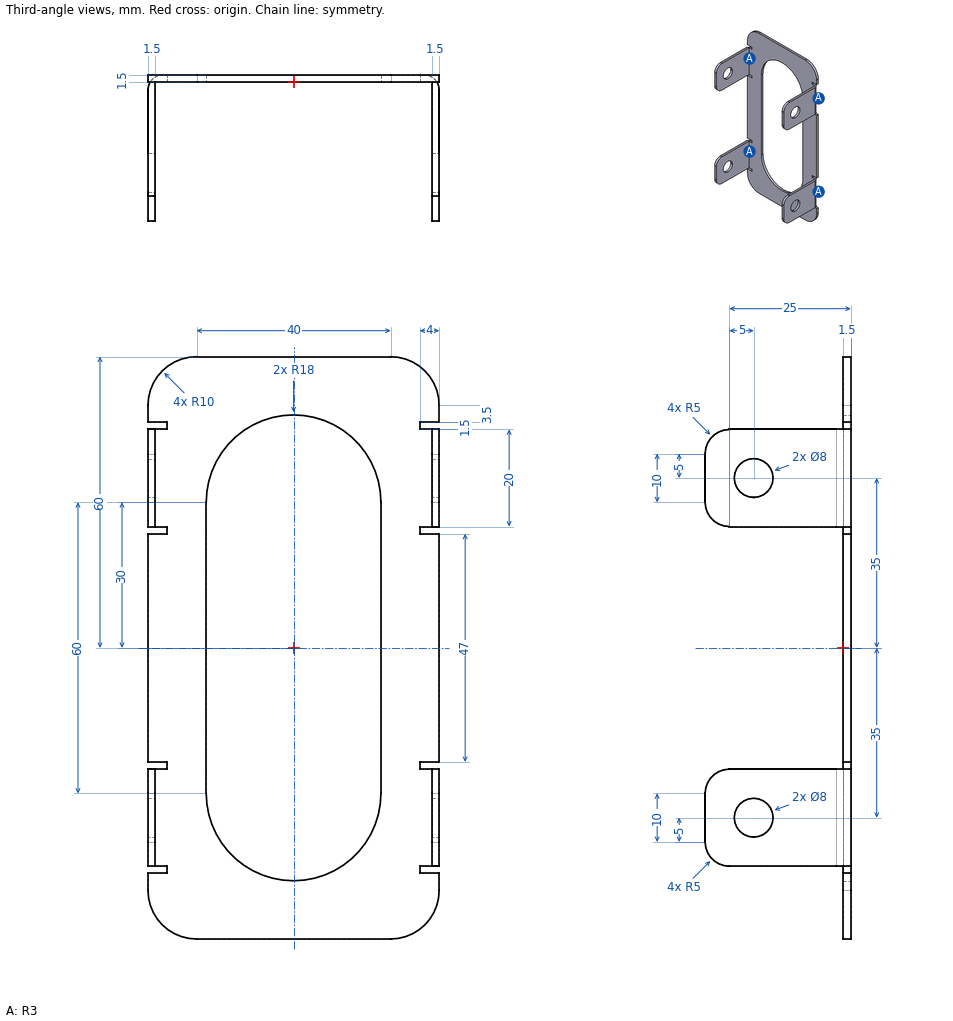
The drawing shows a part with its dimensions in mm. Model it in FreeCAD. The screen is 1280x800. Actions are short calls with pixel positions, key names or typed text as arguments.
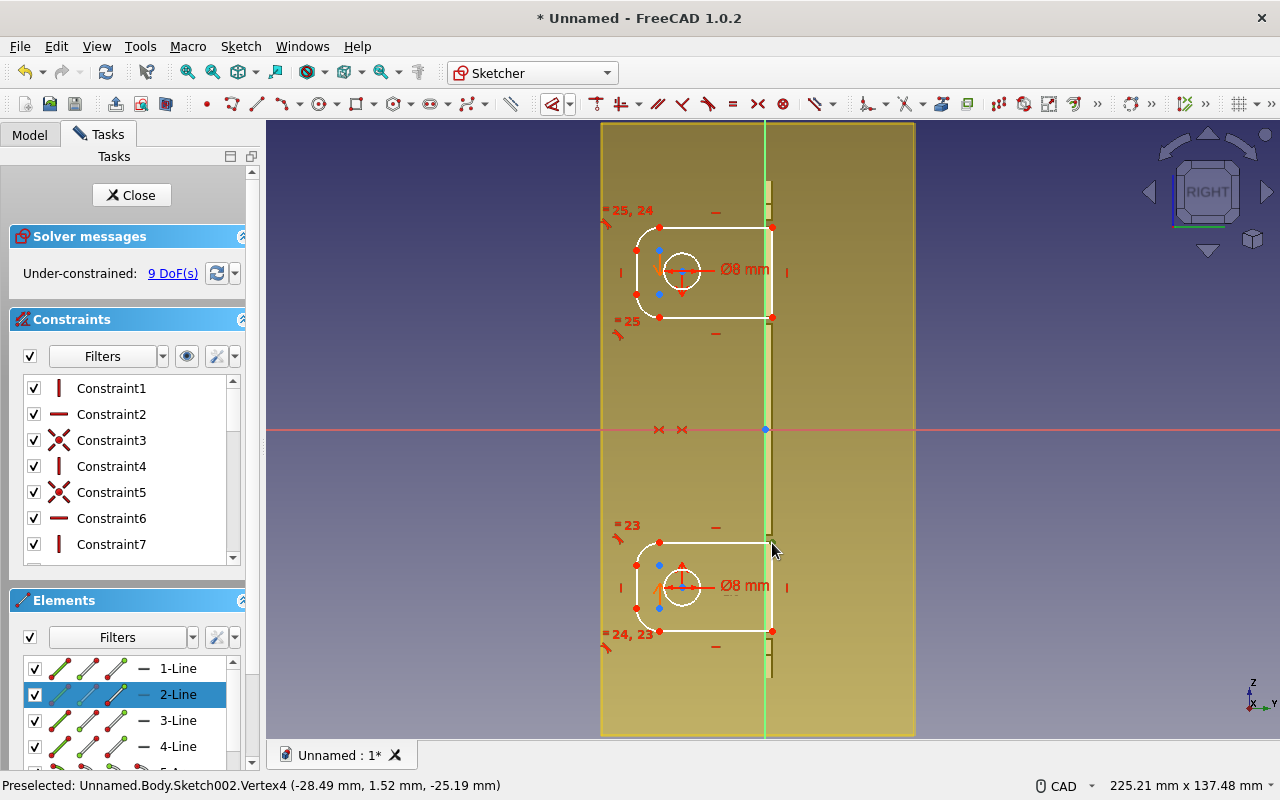
click(772, 318)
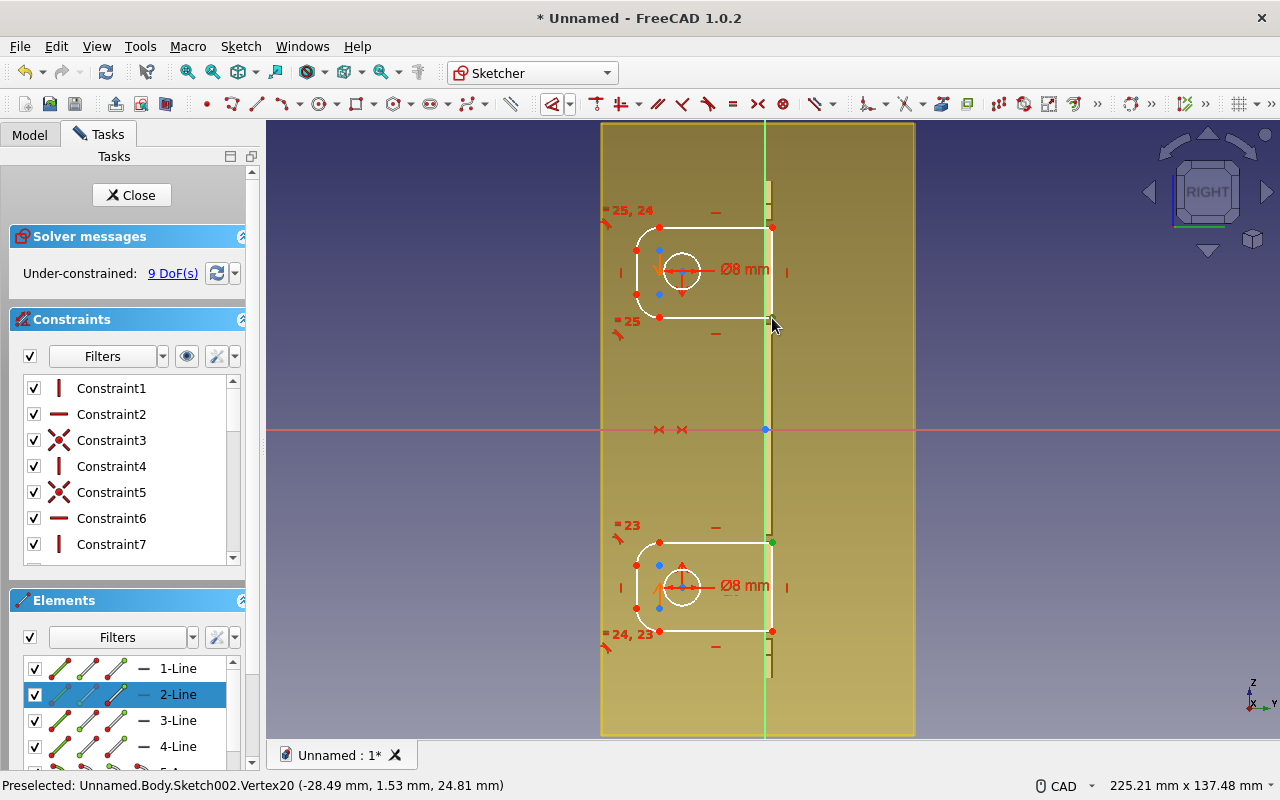
click(353, 430)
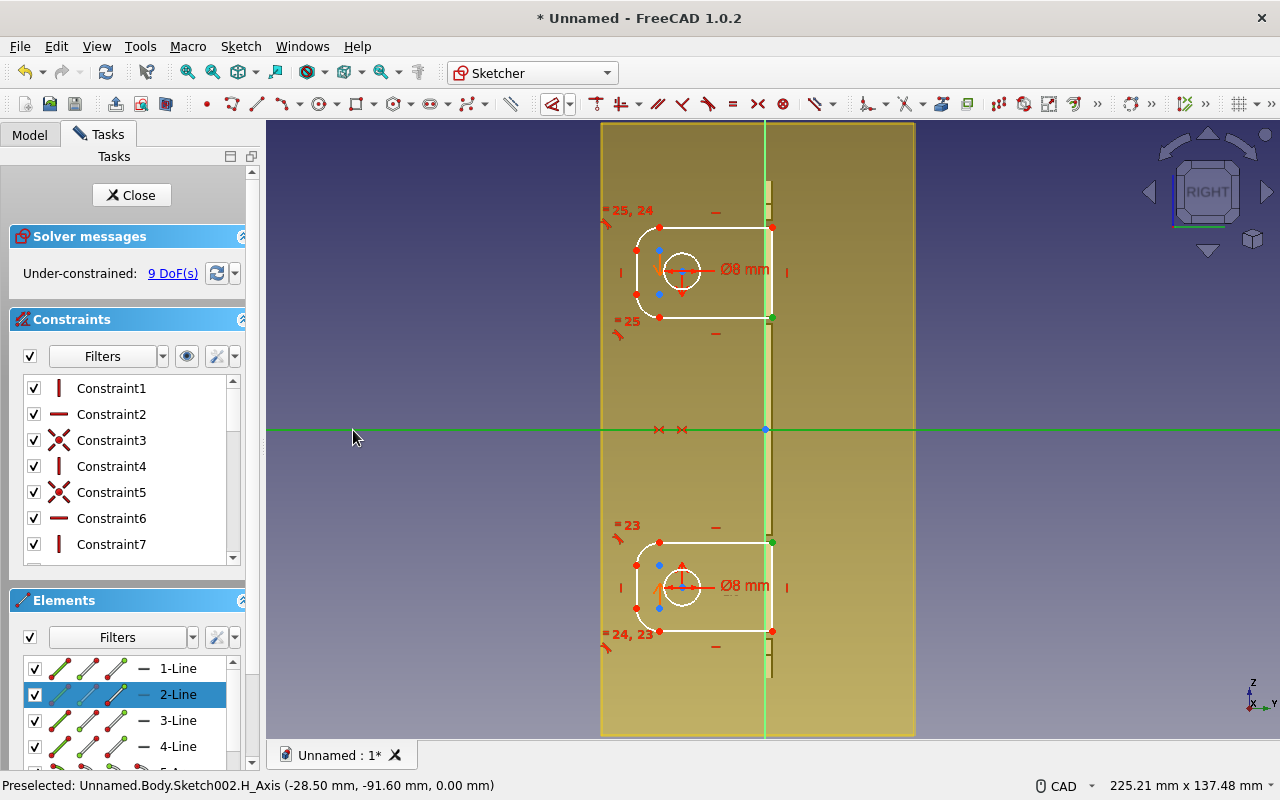
click(758, 104)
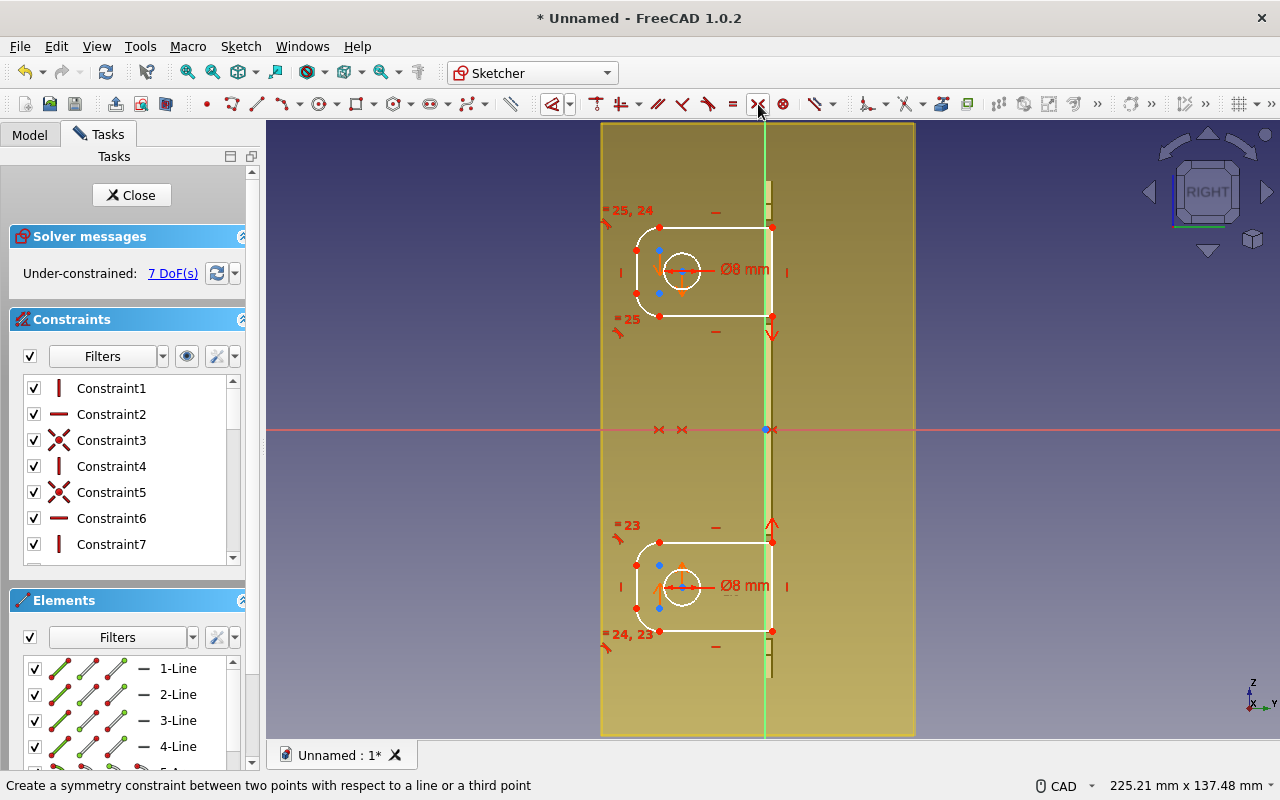
scroll(649, 545, up, 3)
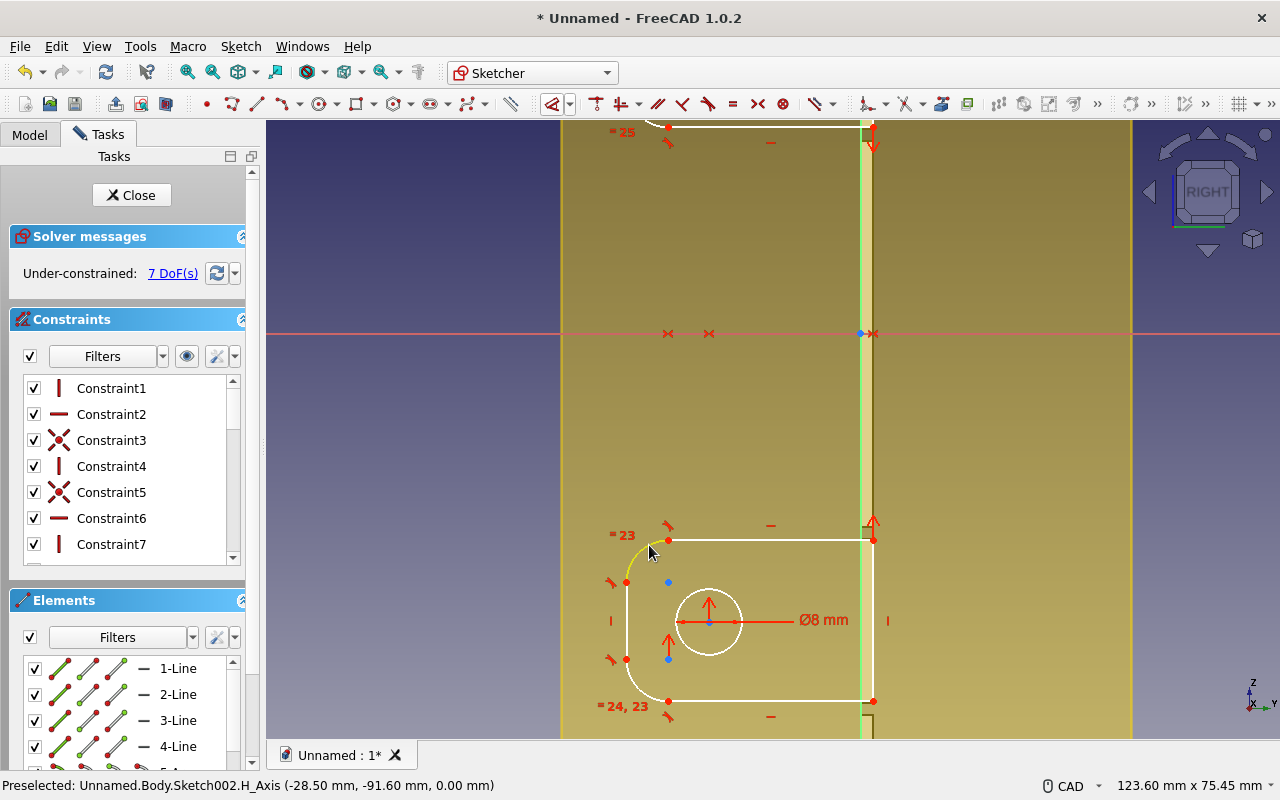
click(650, 545)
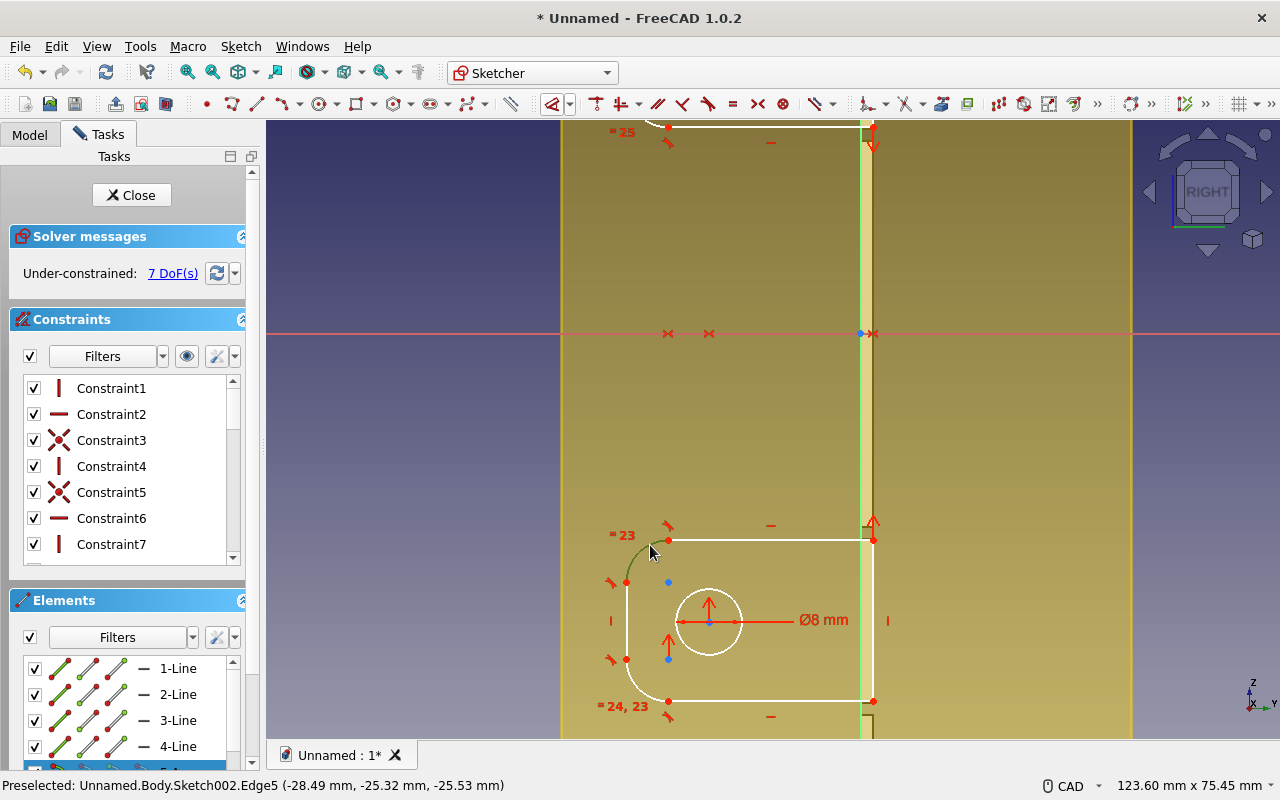
key(k)
key(r)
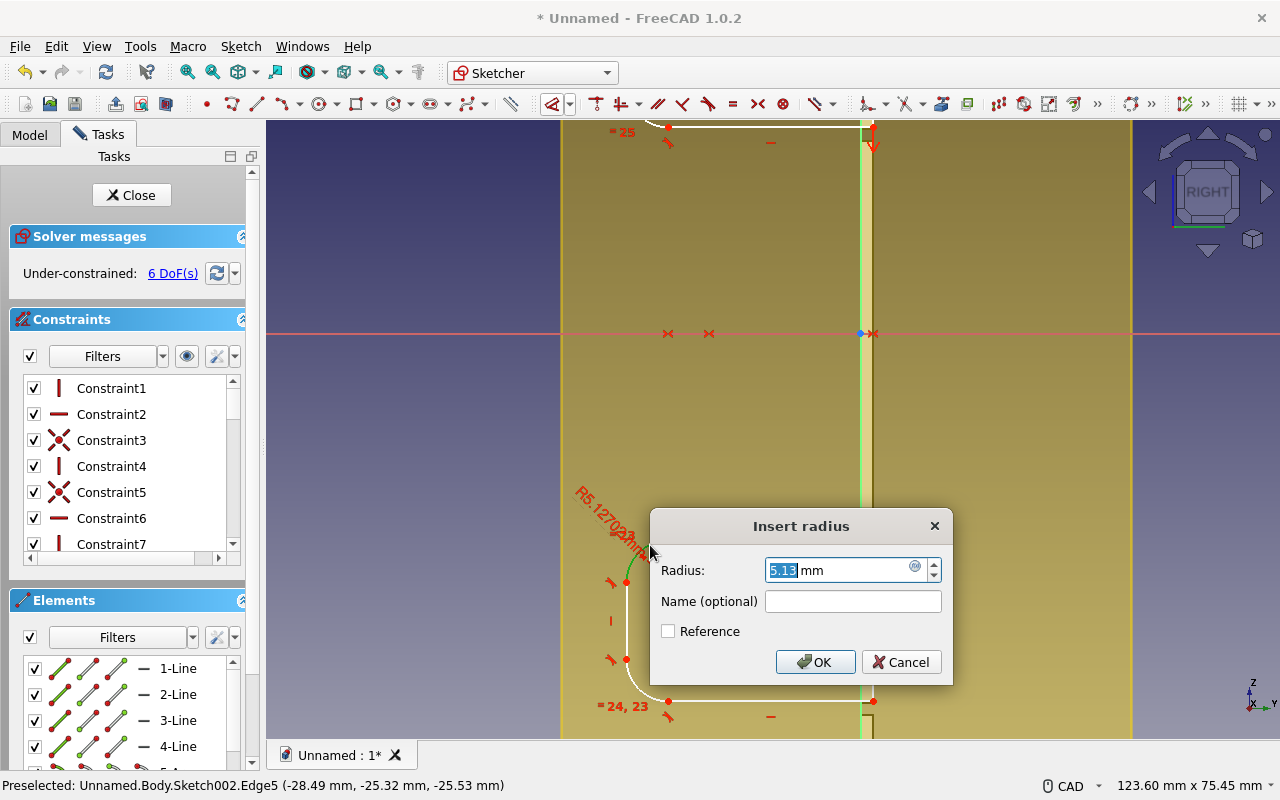
text(5)
key(Return)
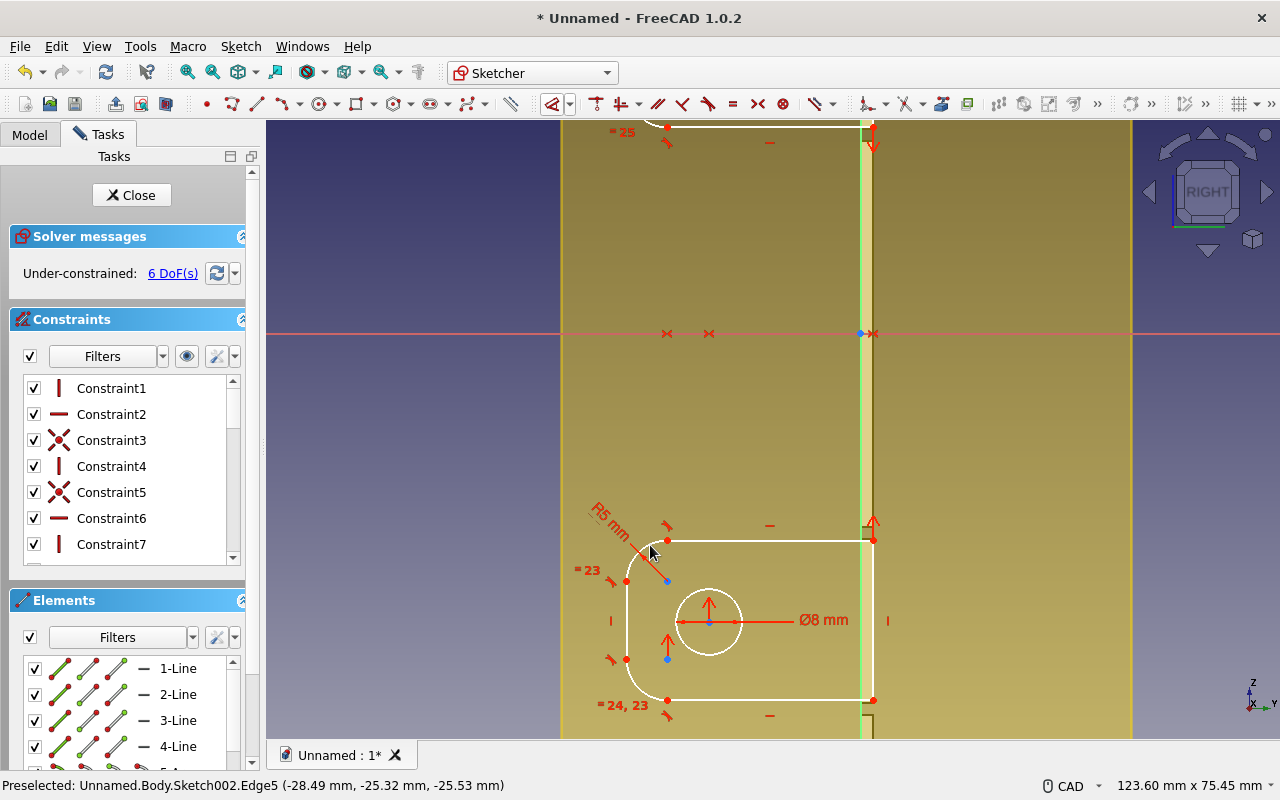
click(627, 636)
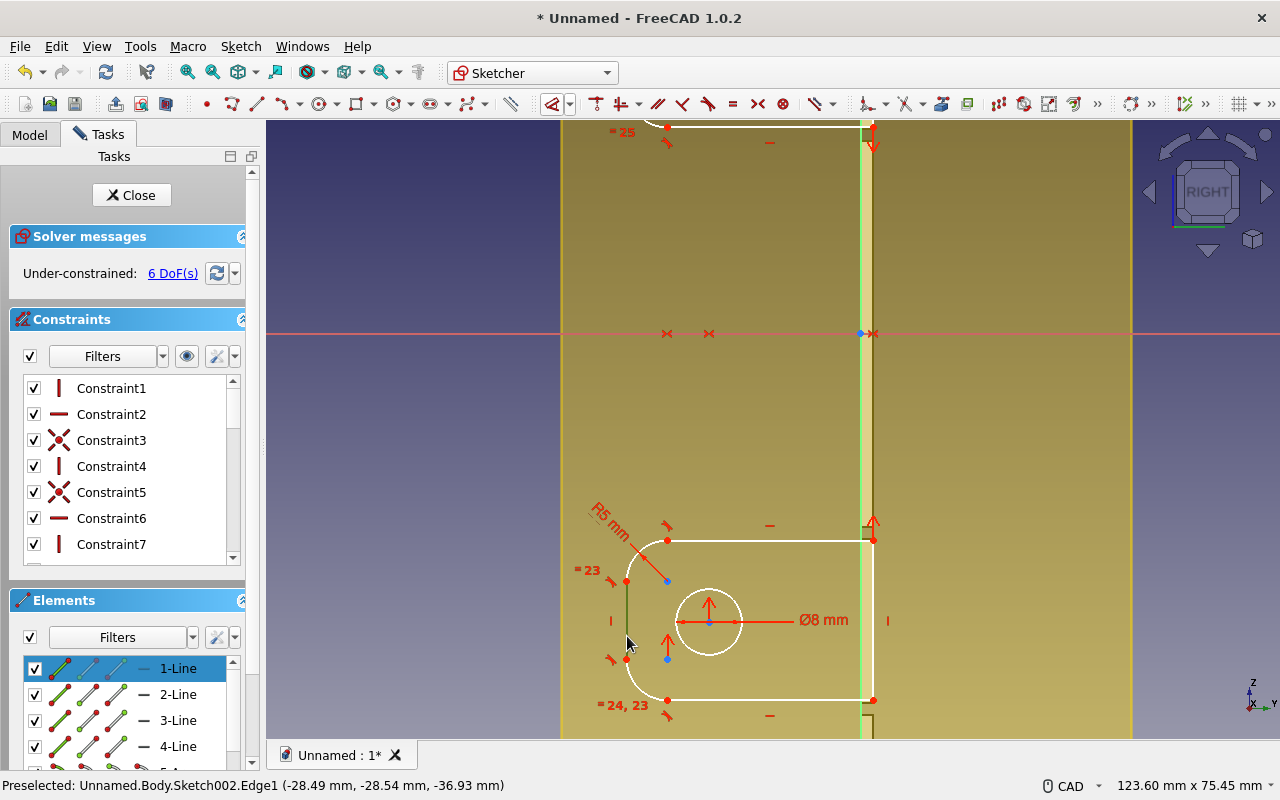
click(570, 104)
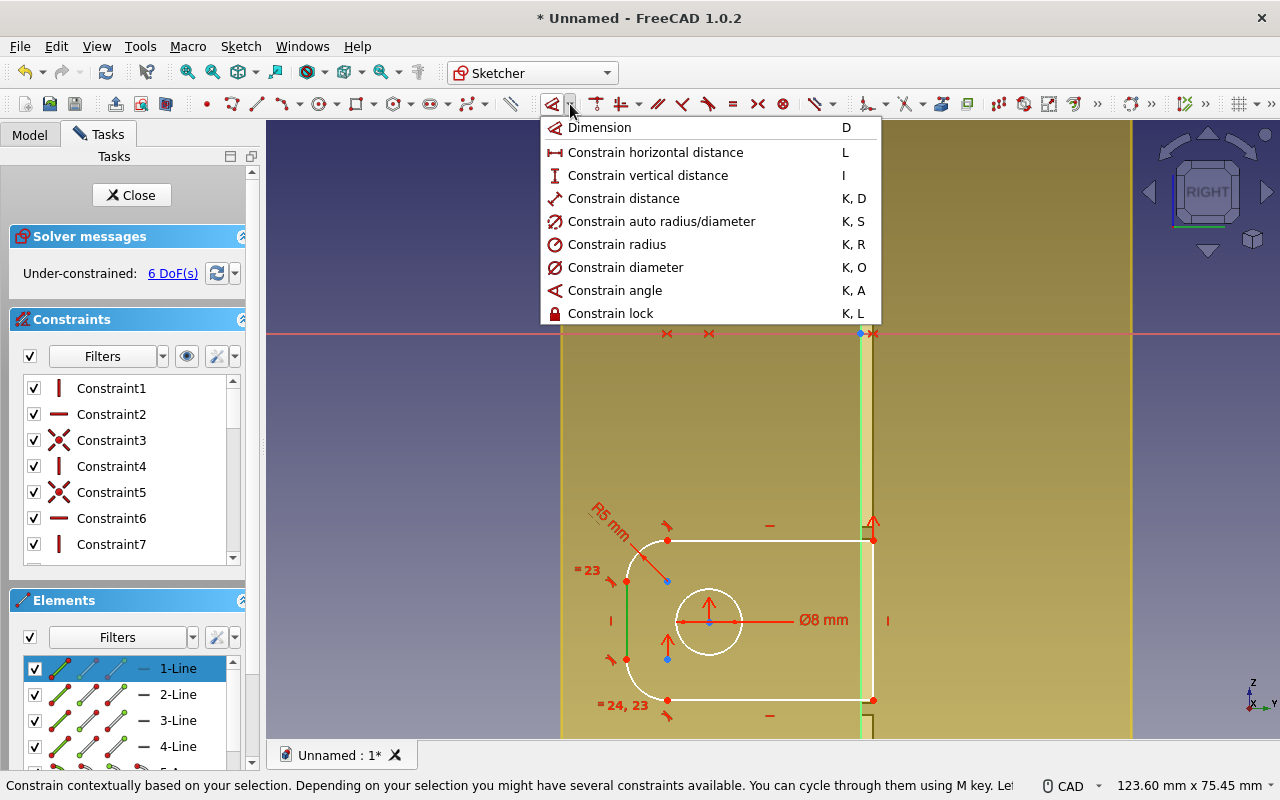
click(711, 176)